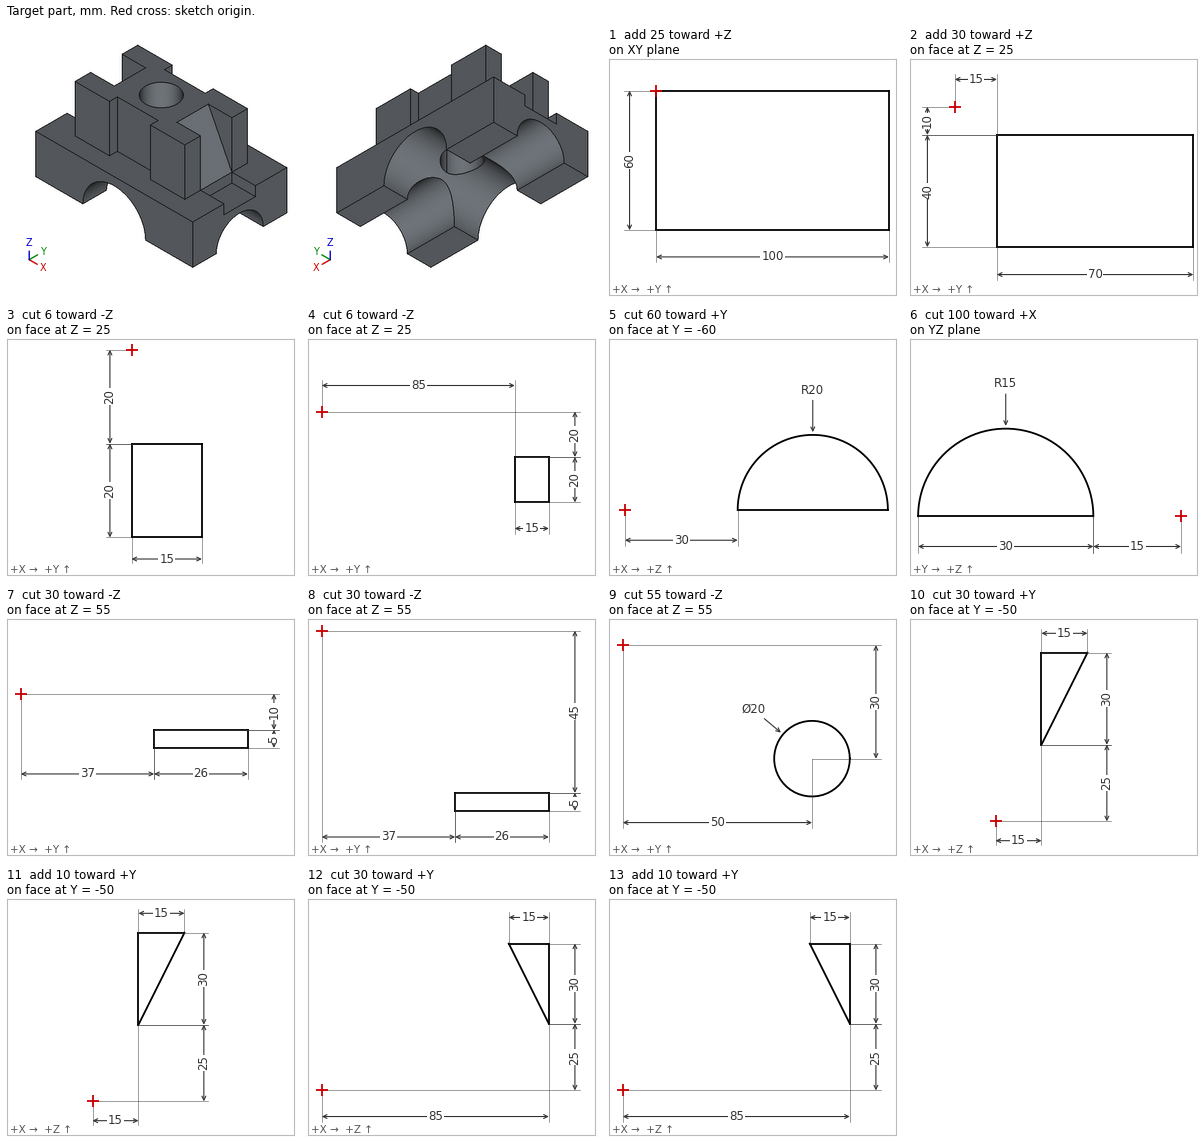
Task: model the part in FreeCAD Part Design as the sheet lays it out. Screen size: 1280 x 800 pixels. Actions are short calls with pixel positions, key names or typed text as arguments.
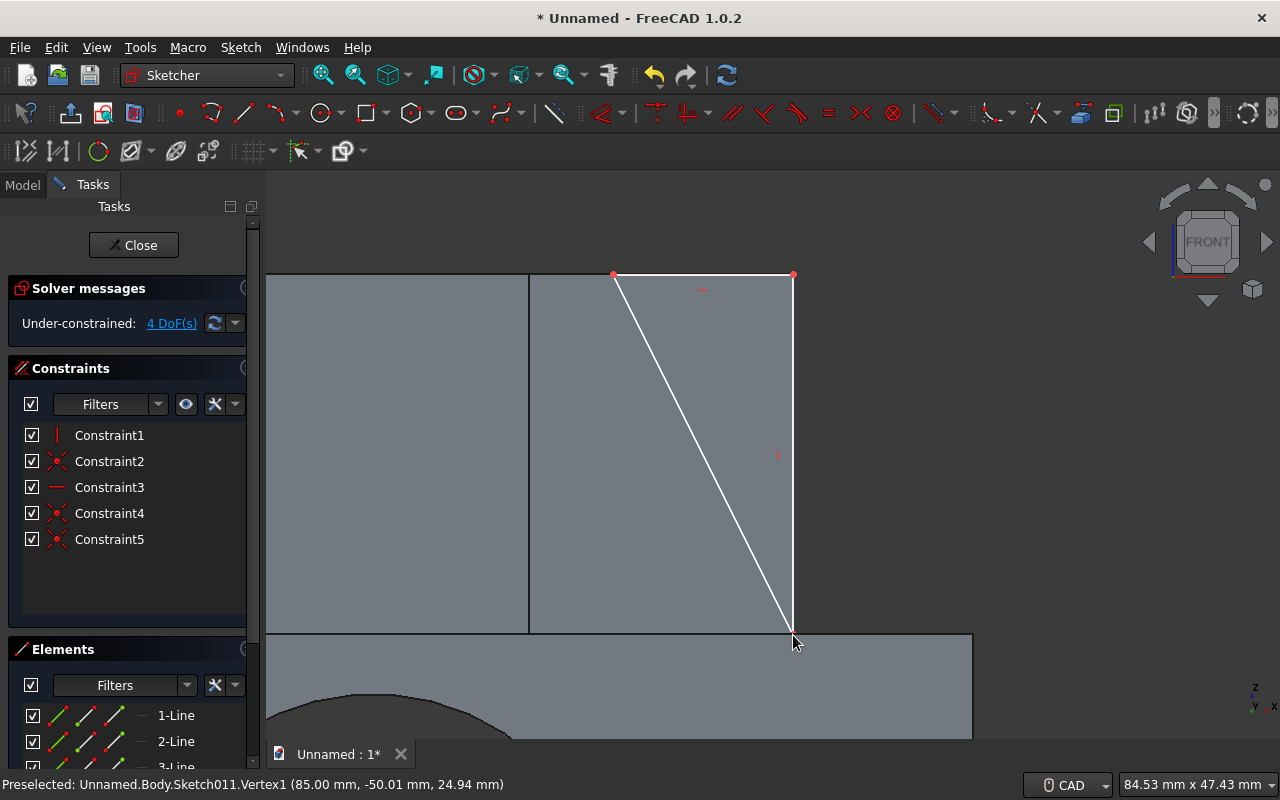
click(602, 114)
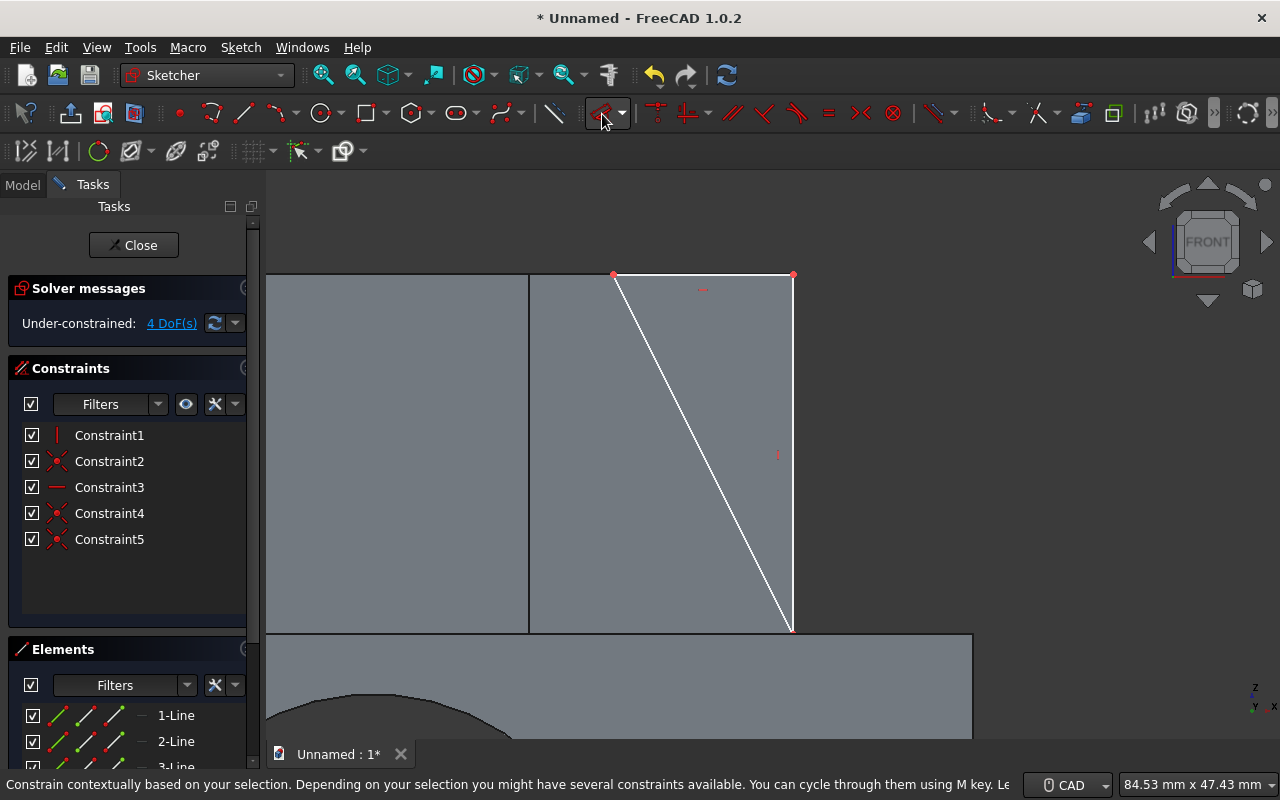
click(793, 527)
click(827, 455)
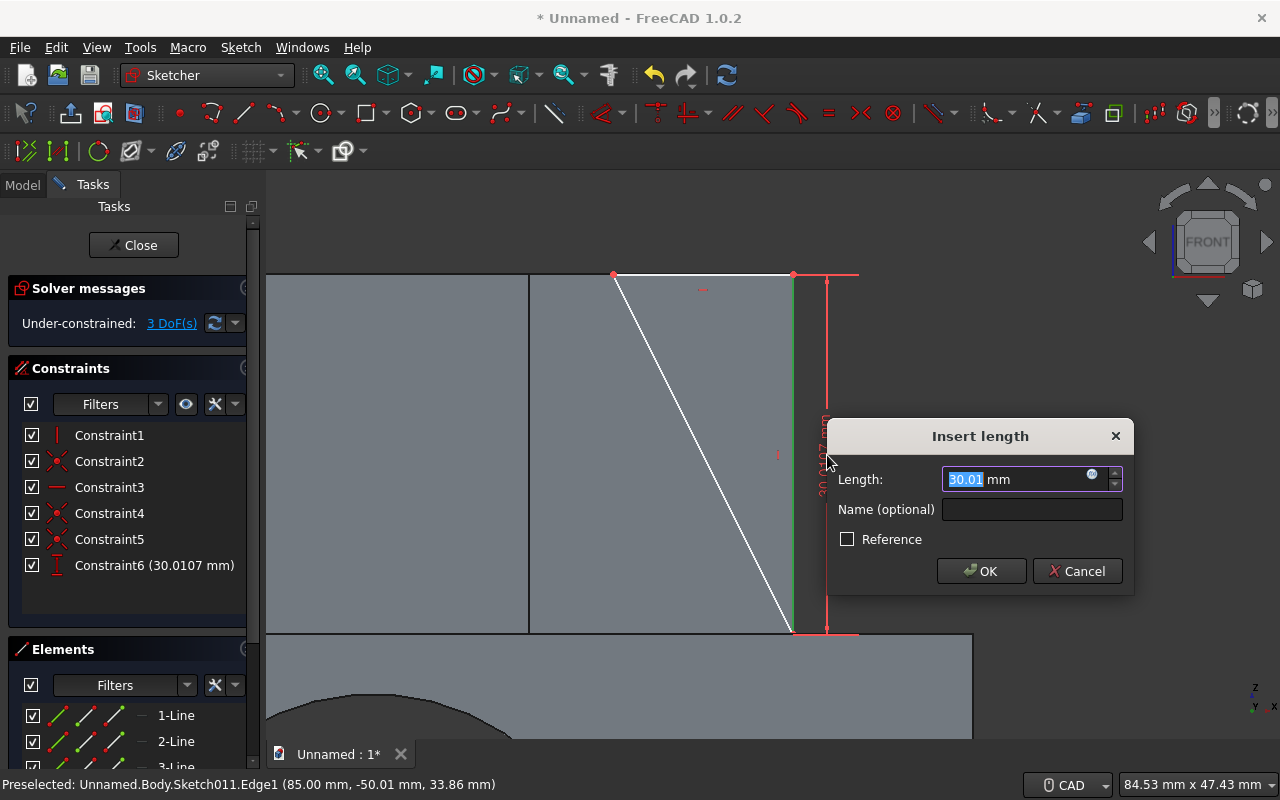
text(30)
key(Return)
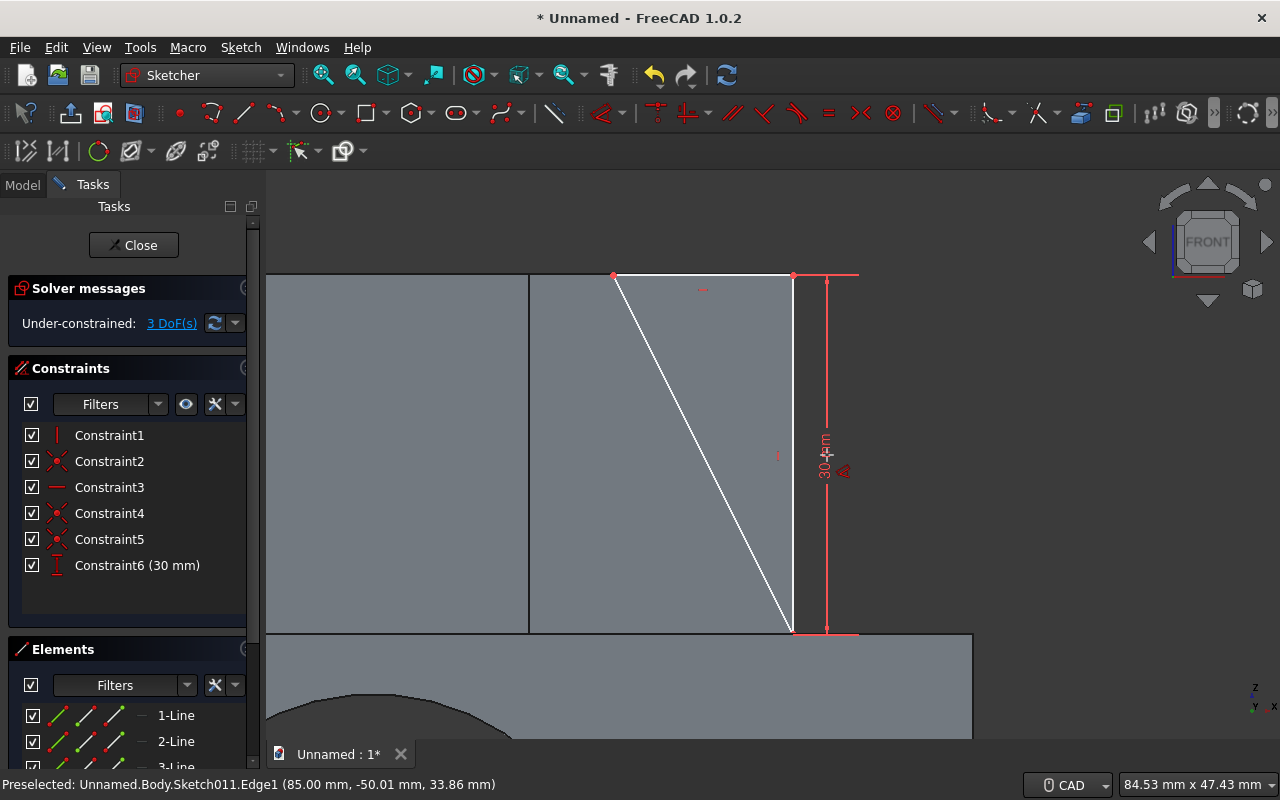
click(739, 275)
click(703, 241)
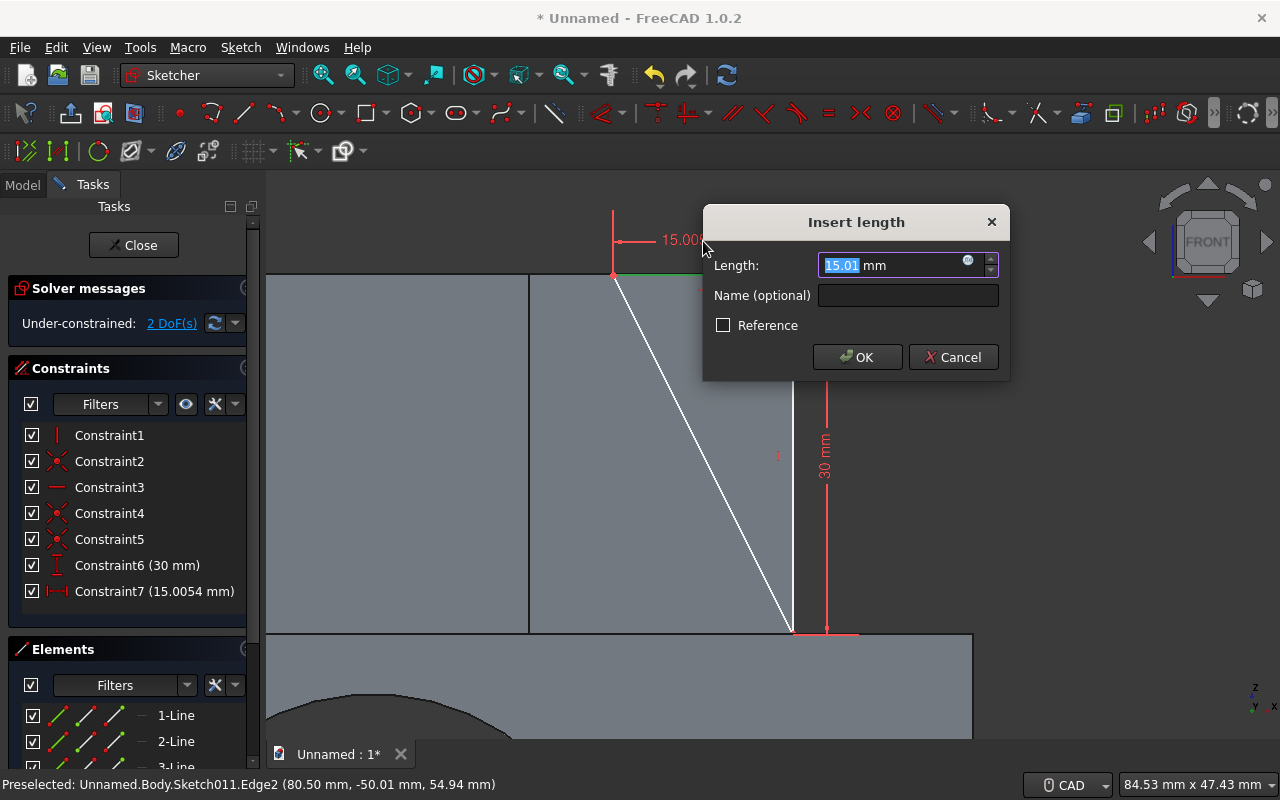
text(15)
key(Return)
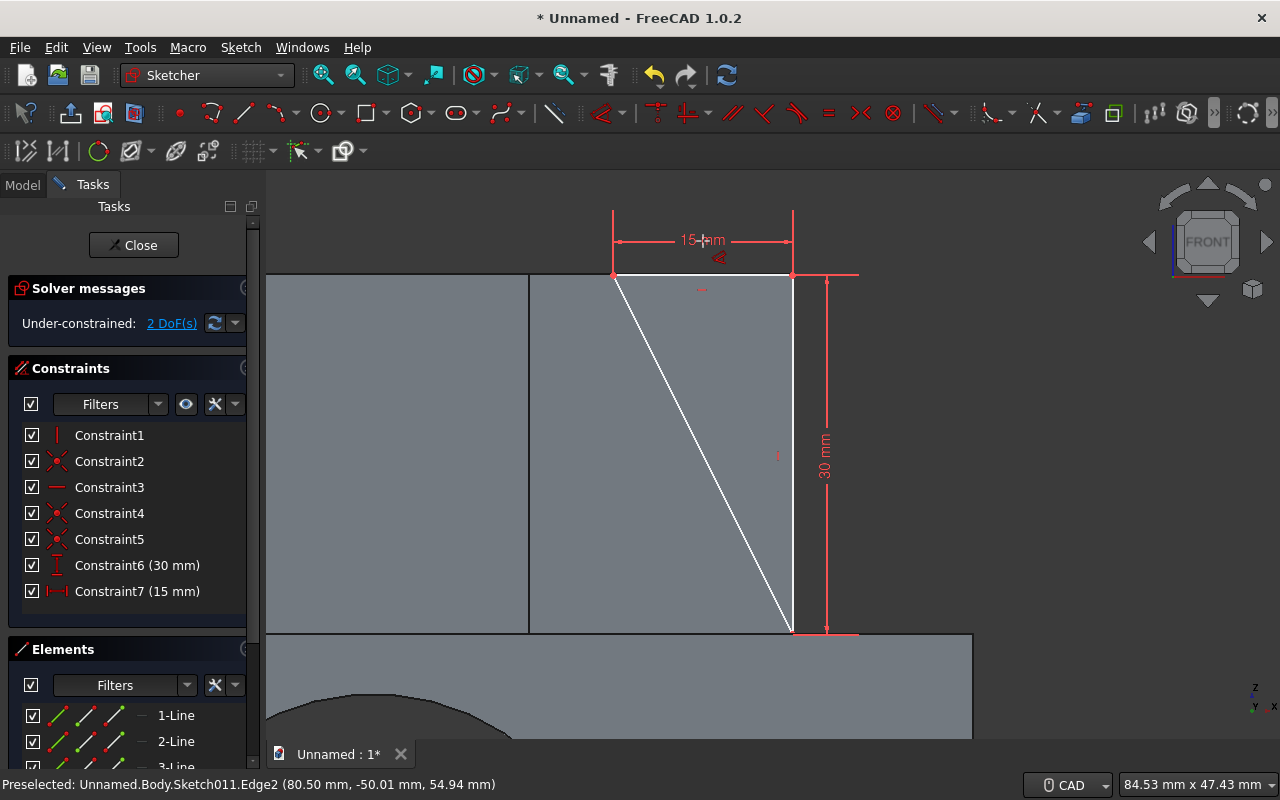
click(793, 635)
click(543, 601)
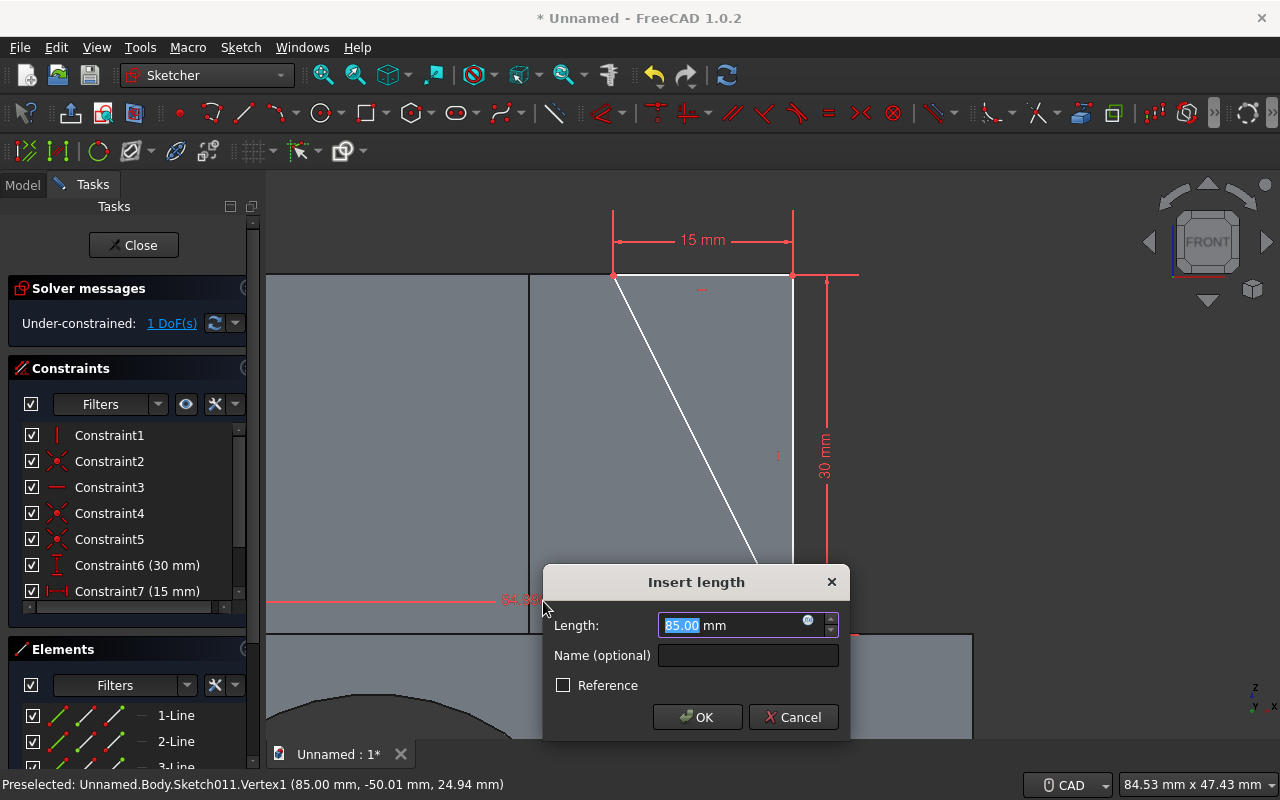
text(85)
key(Return)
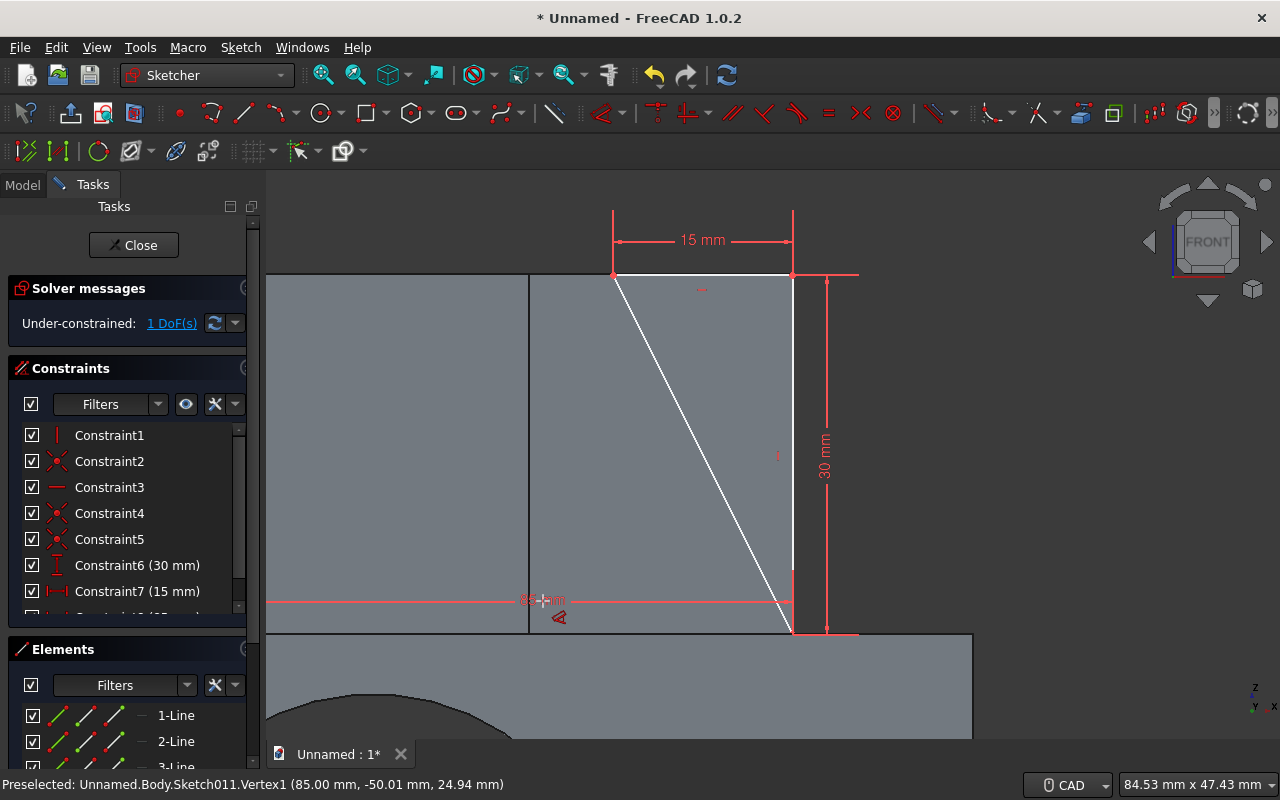
click(793, 635)
click(827, 673)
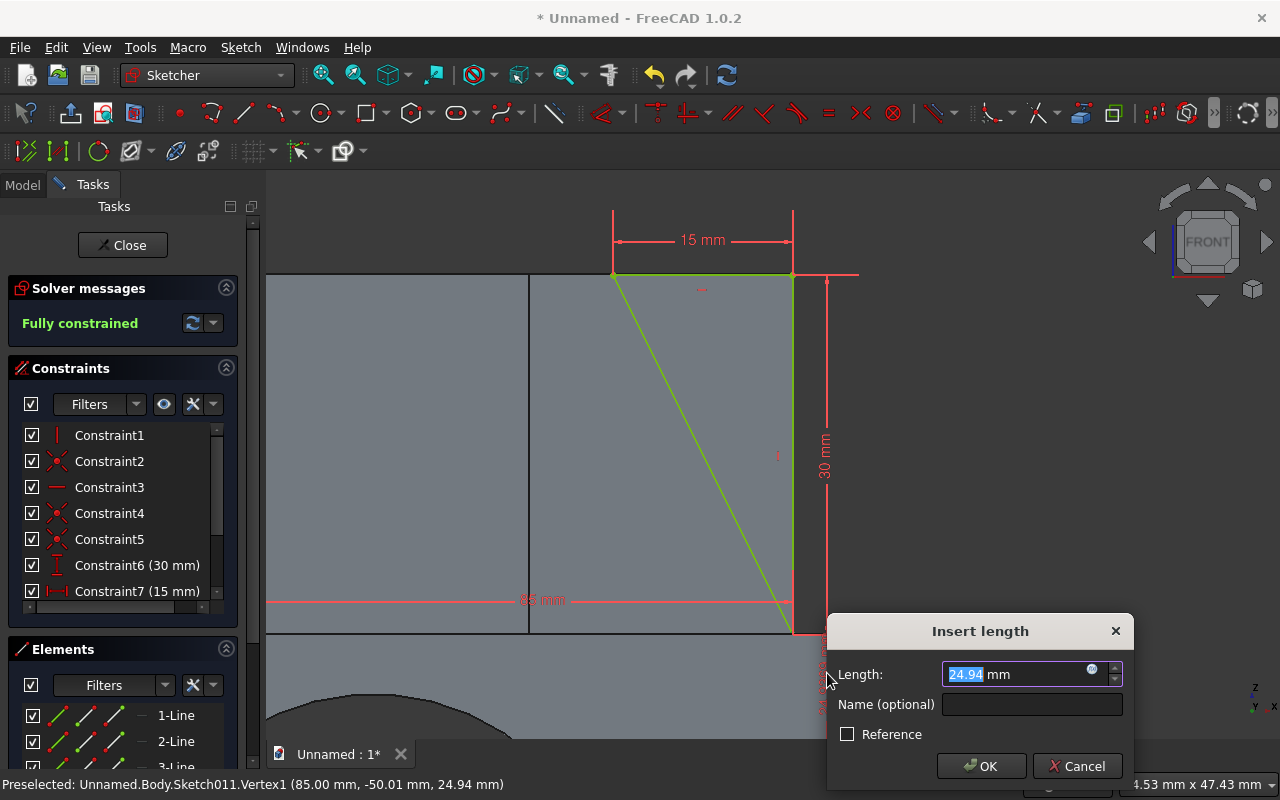
text(25)
key(Return)
key(Escape)